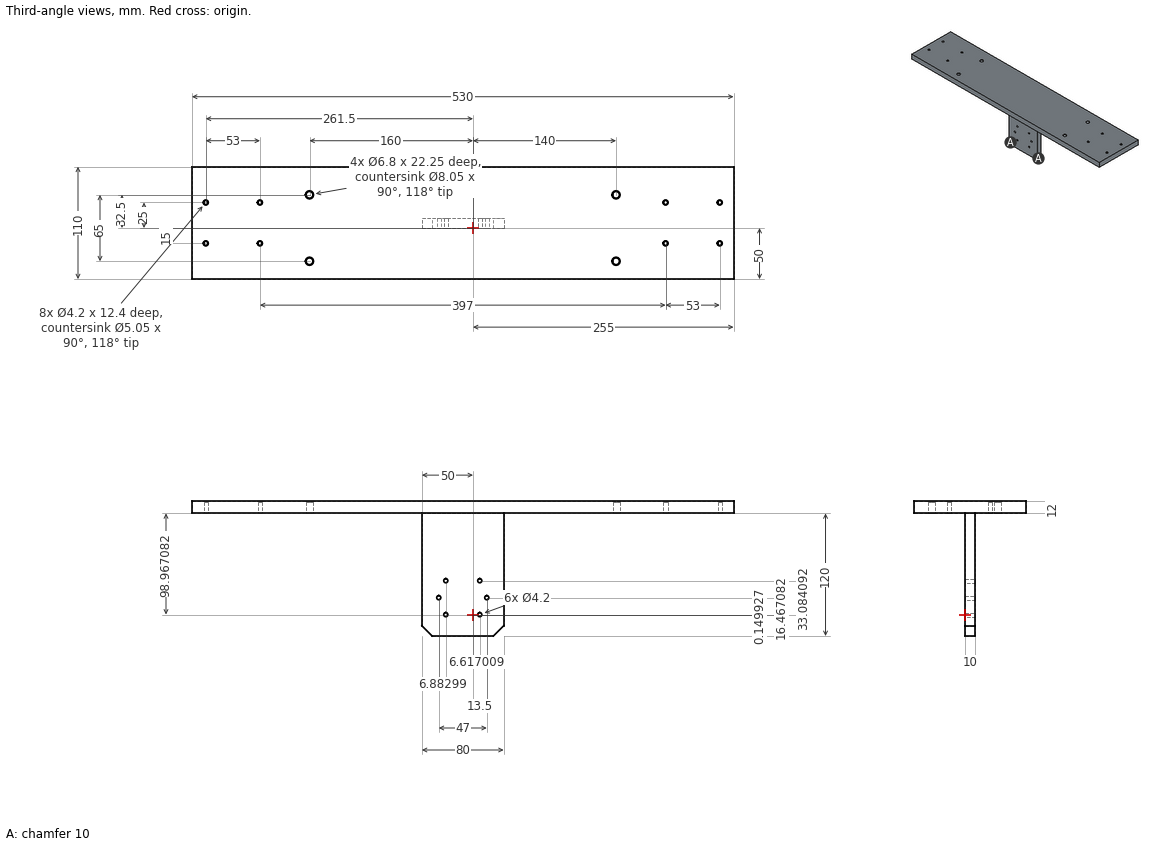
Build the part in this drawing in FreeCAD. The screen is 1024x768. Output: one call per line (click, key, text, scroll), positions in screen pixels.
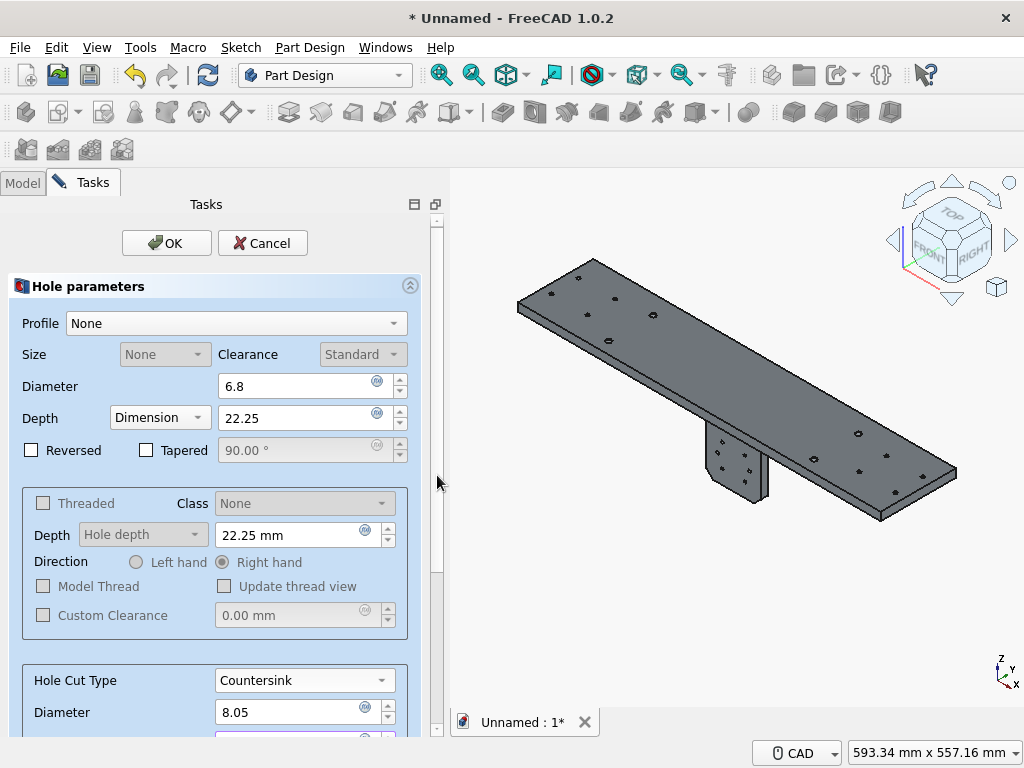
click(167, 243)